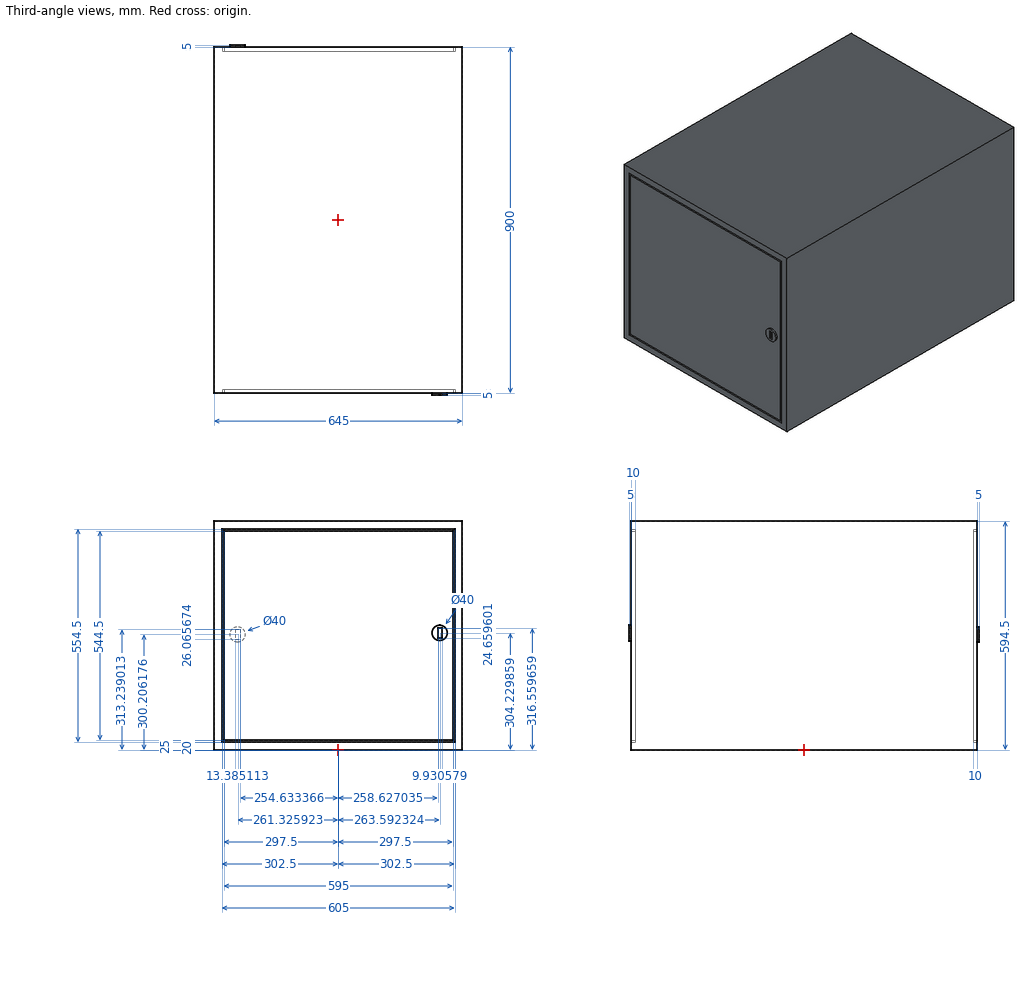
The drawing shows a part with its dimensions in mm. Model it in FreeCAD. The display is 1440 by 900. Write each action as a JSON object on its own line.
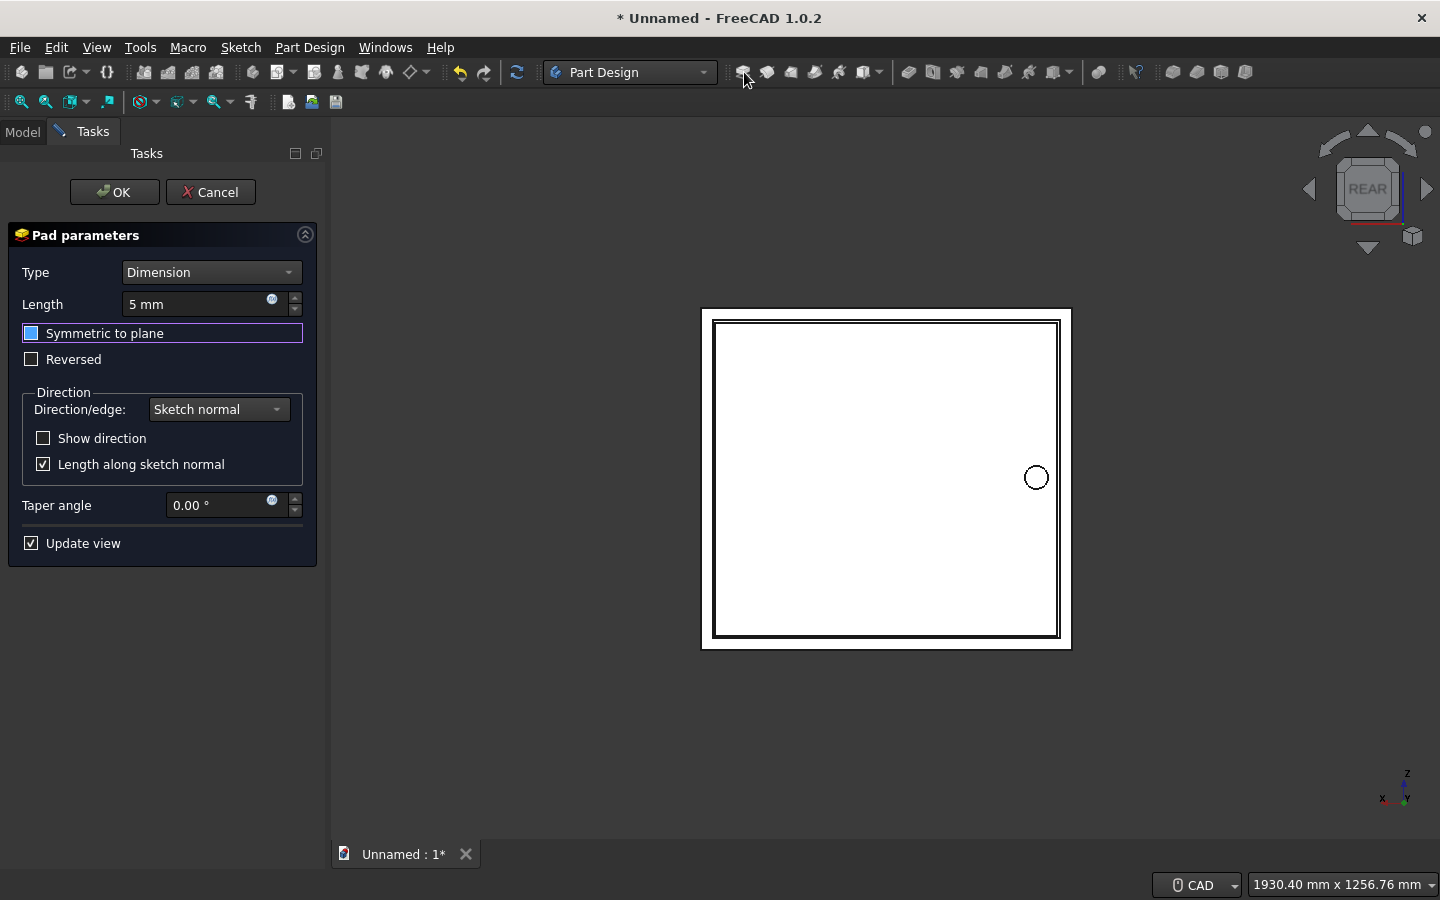
{"action": "left_click", "coordinate": [115, 192]}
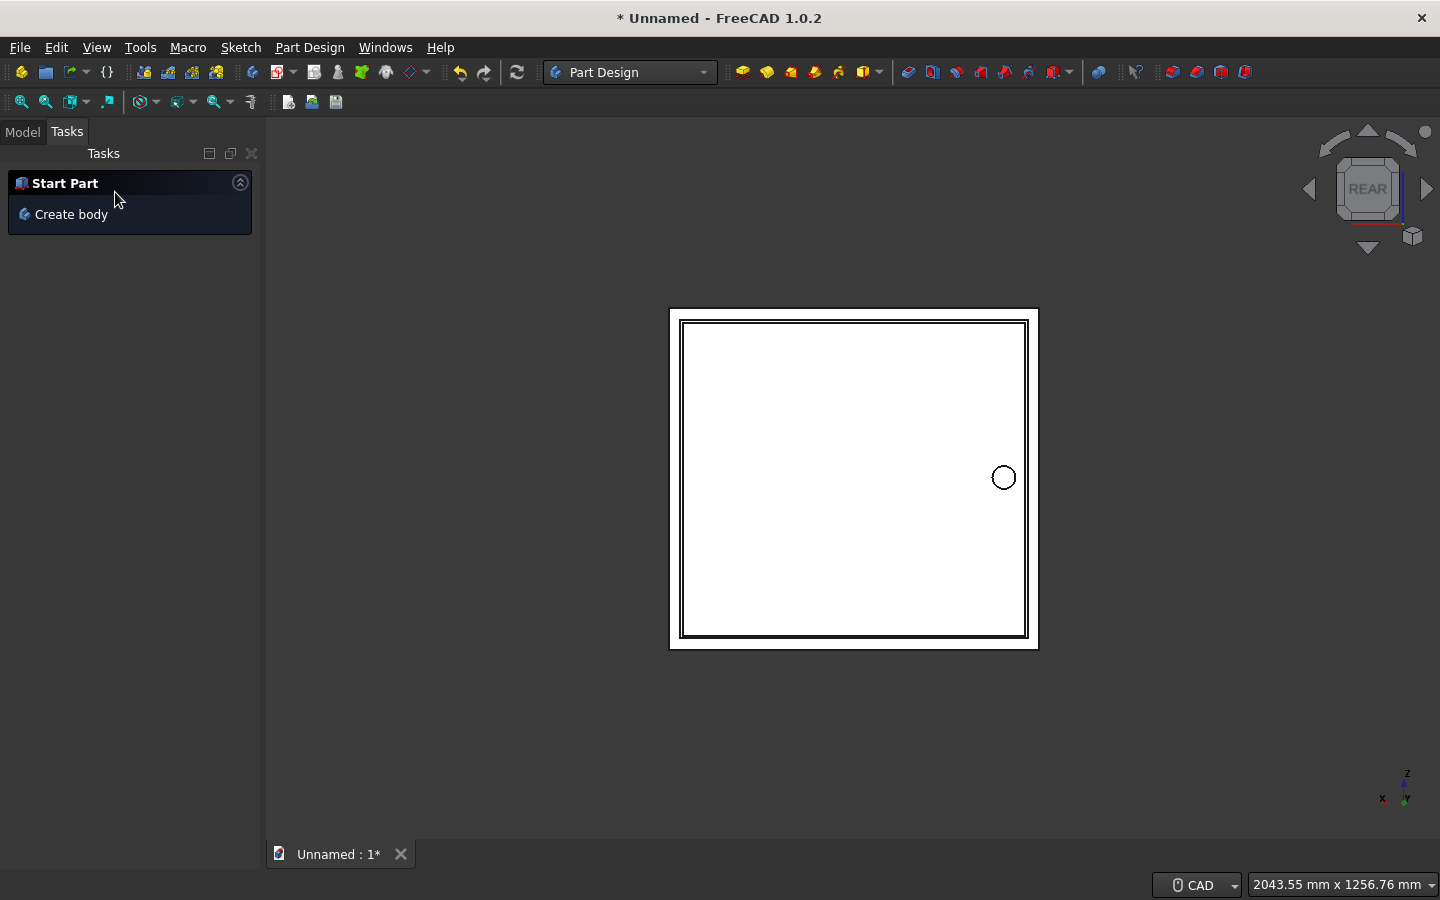
{"action": "left_click", "coordinate": [1004, 476]}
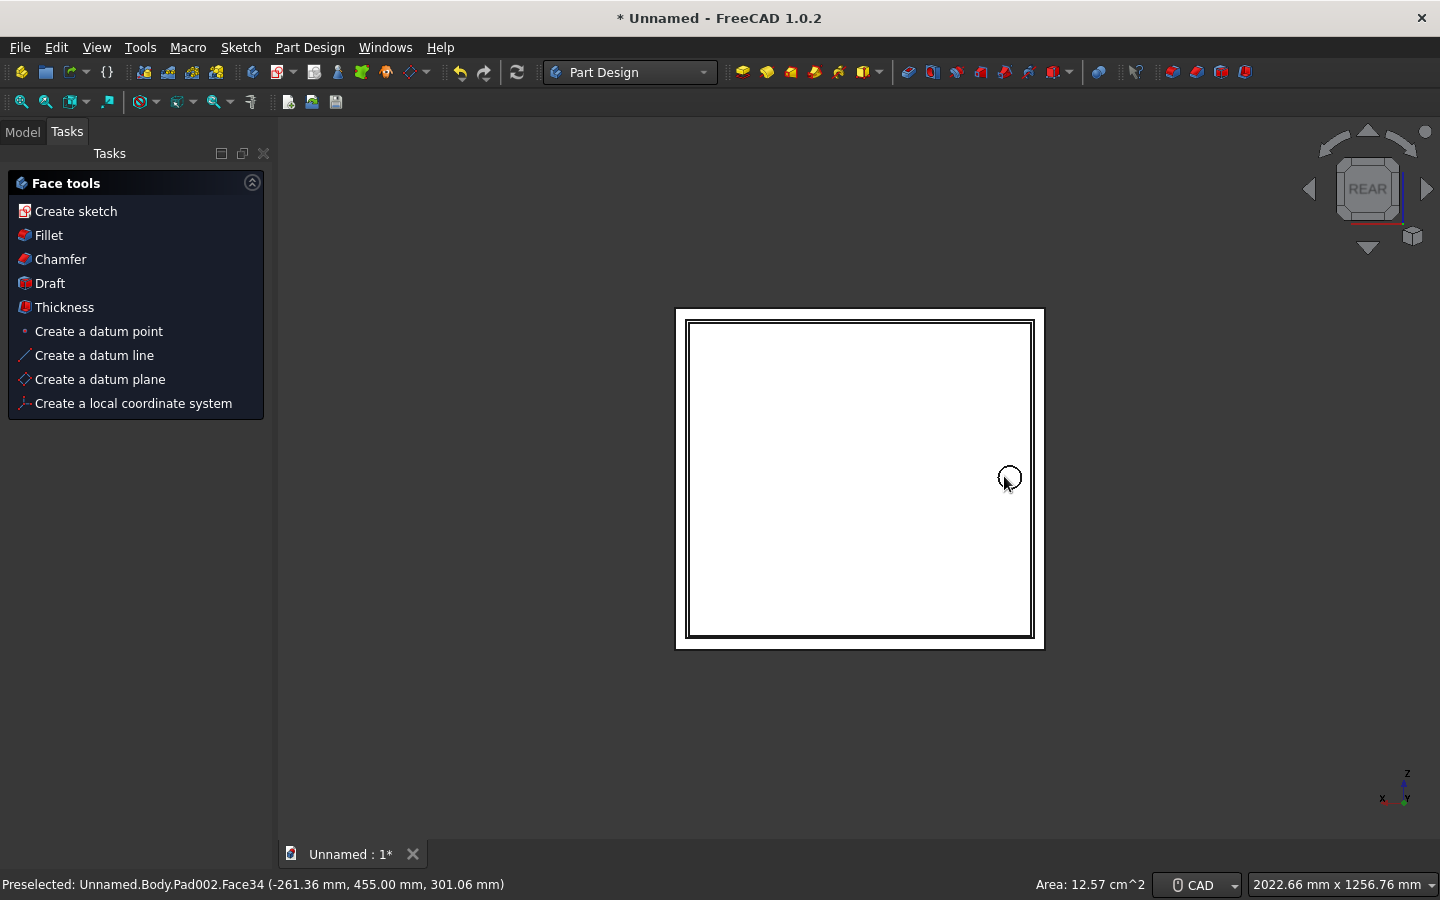
{"action": "left_click", "coordinate": [278, 72]}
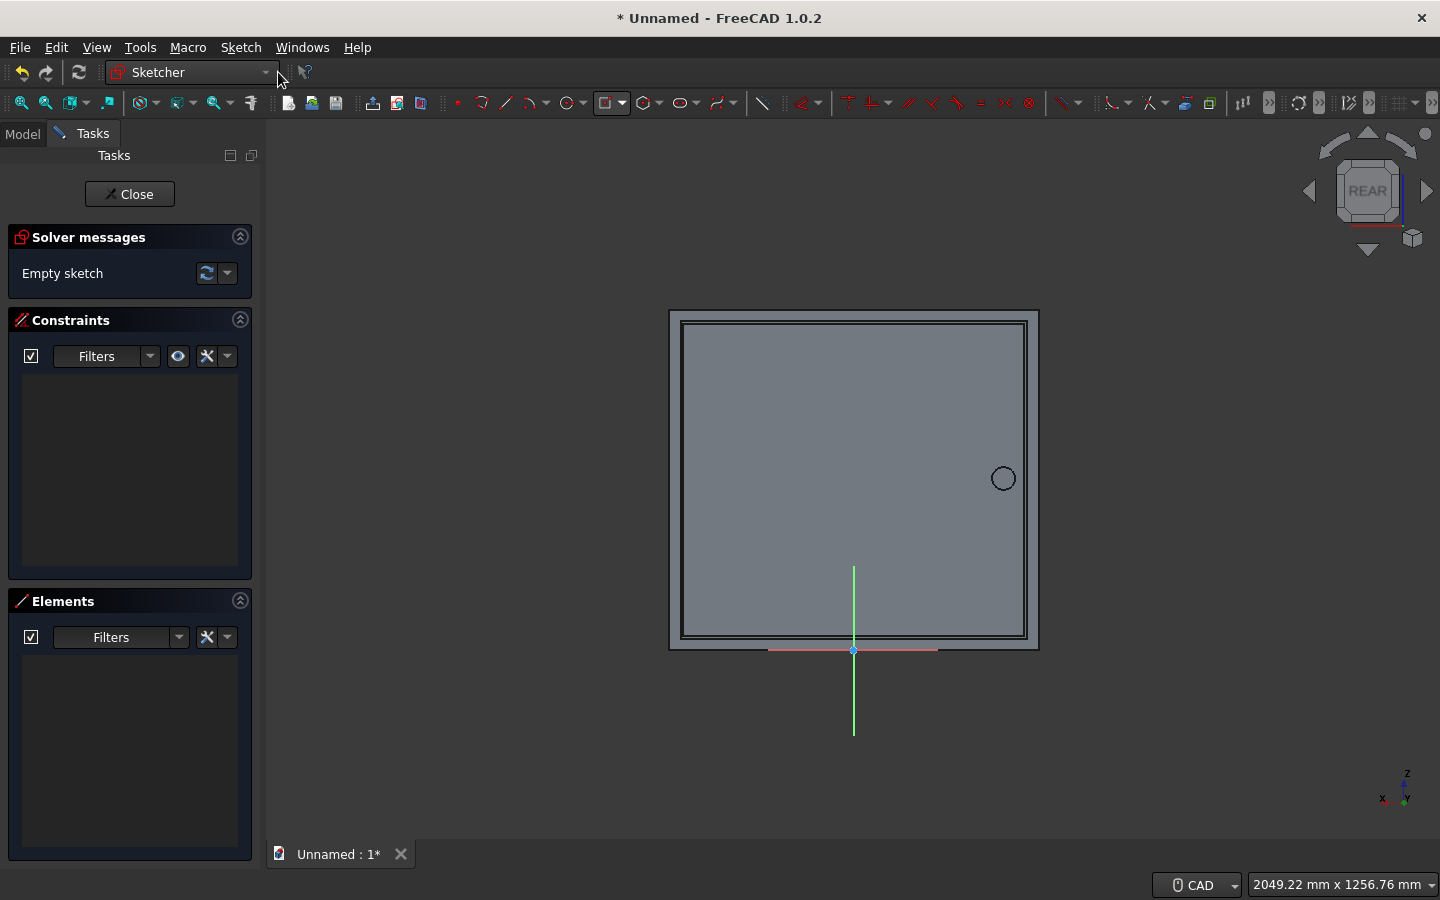
{"action": "scroll", "coordinate": [1015, 478], "scroll_direction": "up", "scroll_amount": 15}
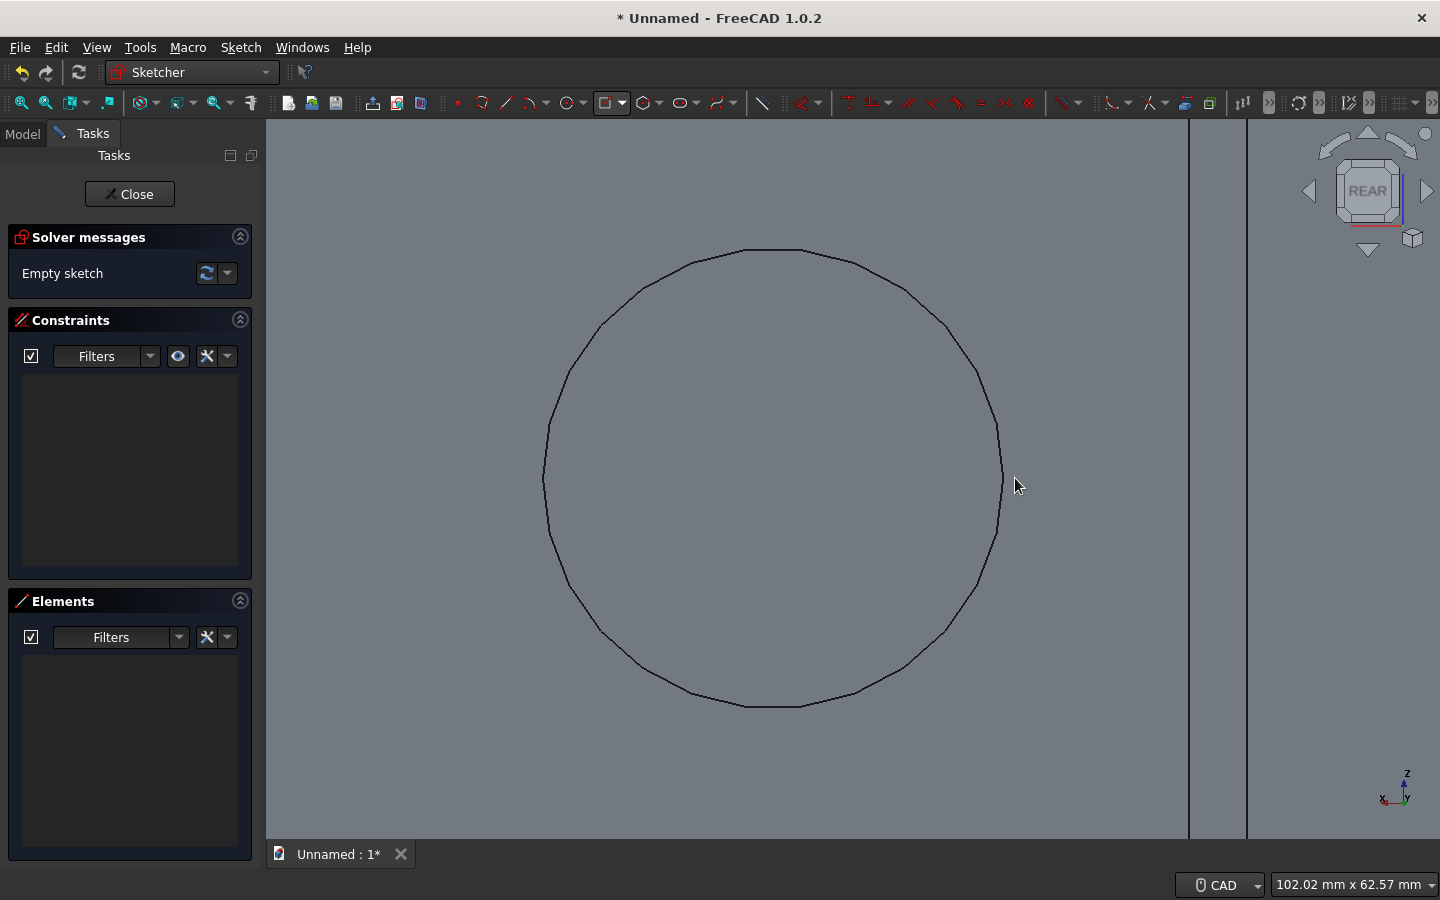
{"action": "scroll", "coordinate": [750, 477], "scroll_direction": "up", "scroll_amount": 2}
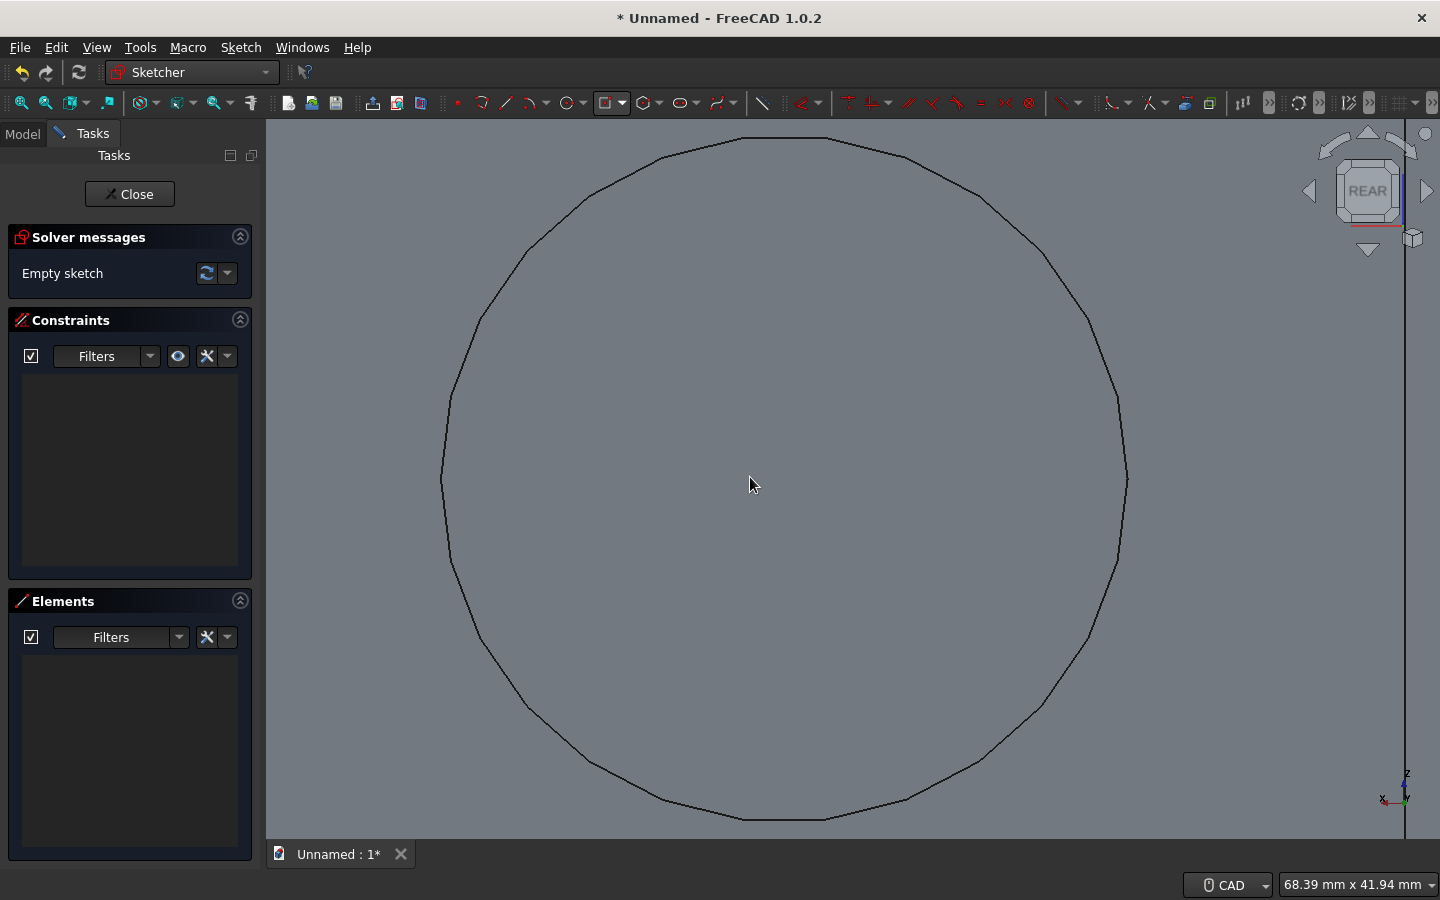
{"action": "key", "text": "g r"}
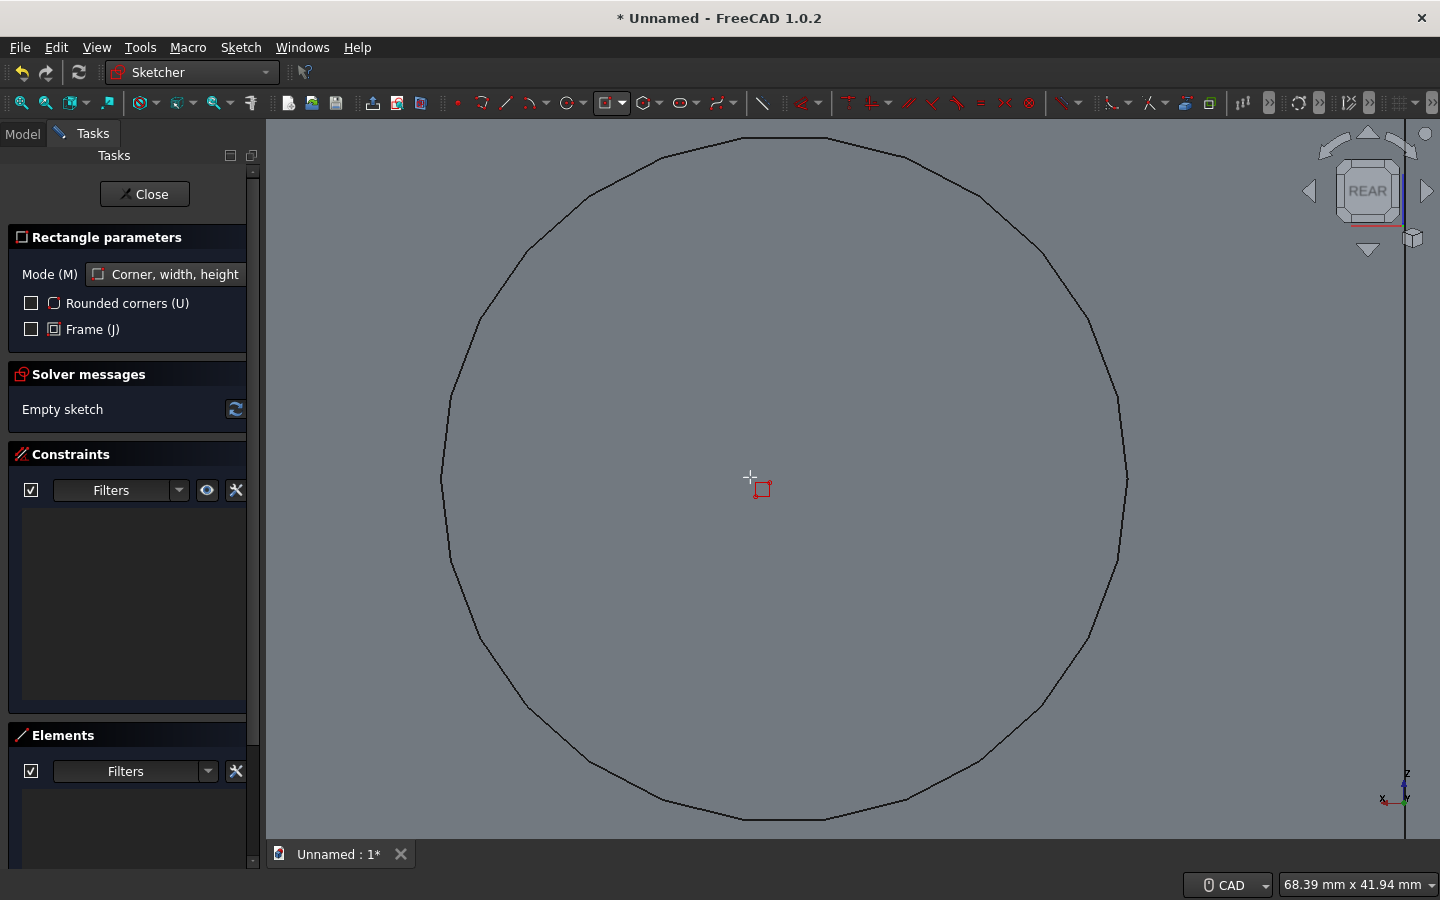
{"action": "left_click", "coordinate": [669, 255]}
{"action": "left_click", "coordinate": [899, 703]}
{"action": "key", "text": "Escape"}